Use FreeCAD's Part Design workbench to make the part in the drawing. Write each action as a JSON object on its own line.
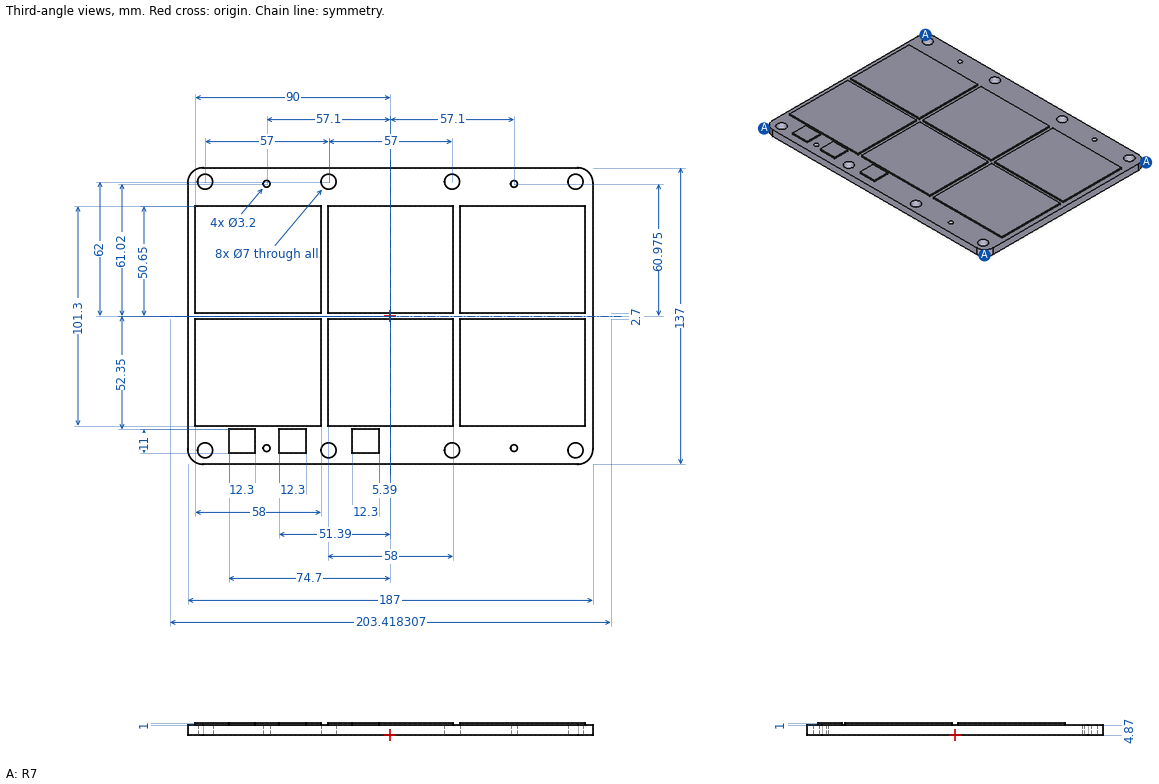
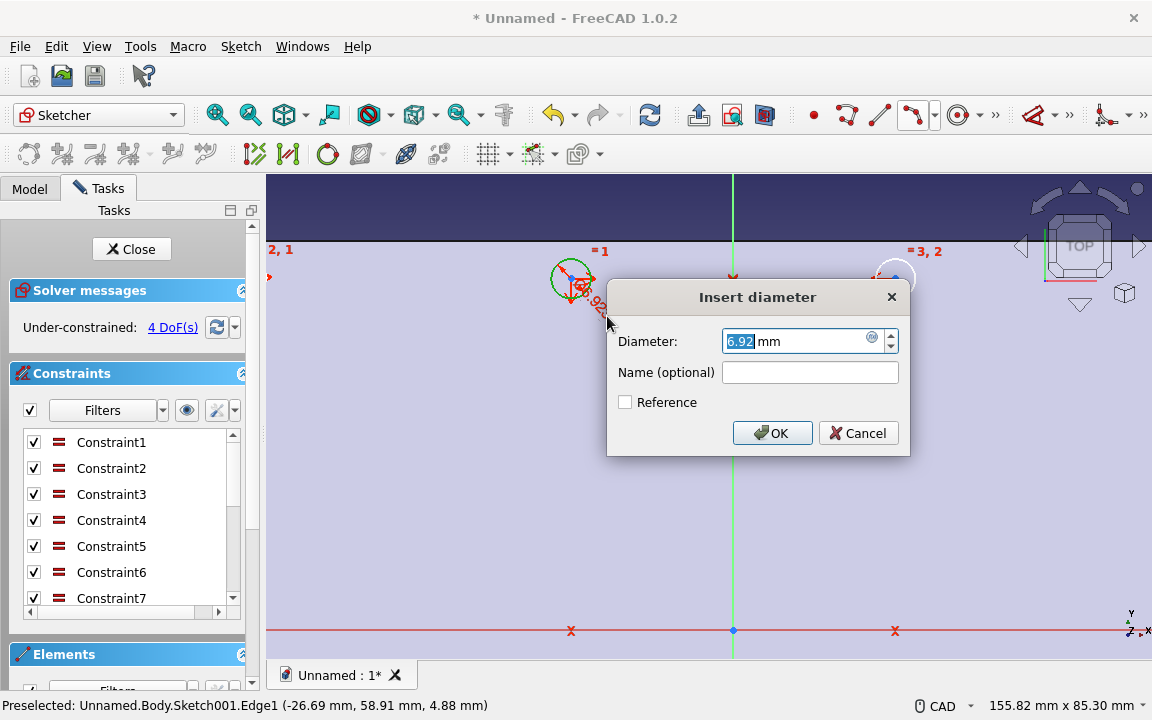
{"action": "type", "text": "7"}
{"action": "key", "text": "Return"}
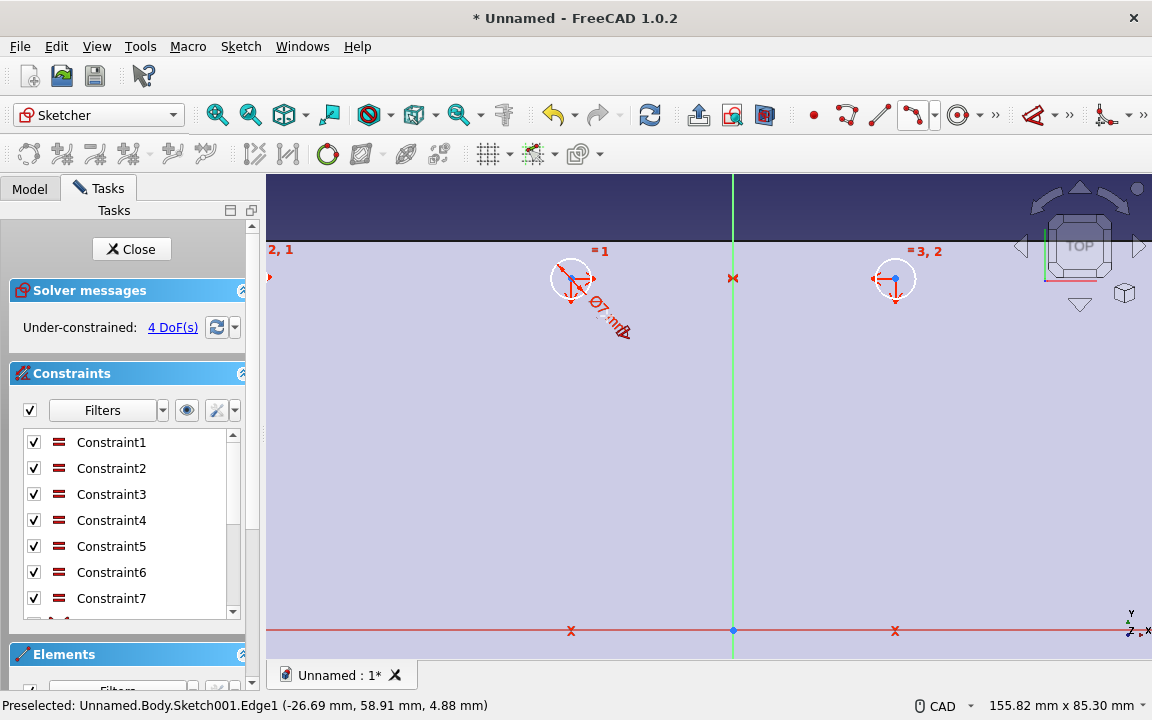
{"action": "left_click", "coordinate": [571, 279]}
{"action": "left_click", "coordinate": [537, 455]}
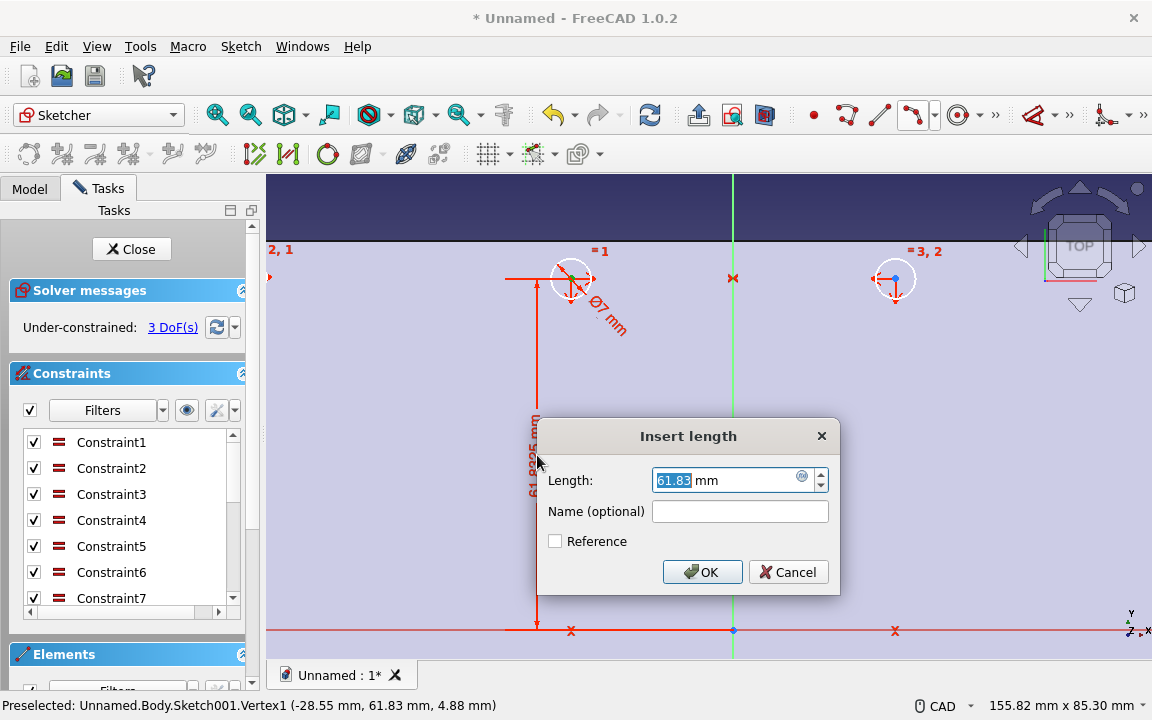
{"action": "type", "text": "62"}
{"action": "key", "text": "Return"}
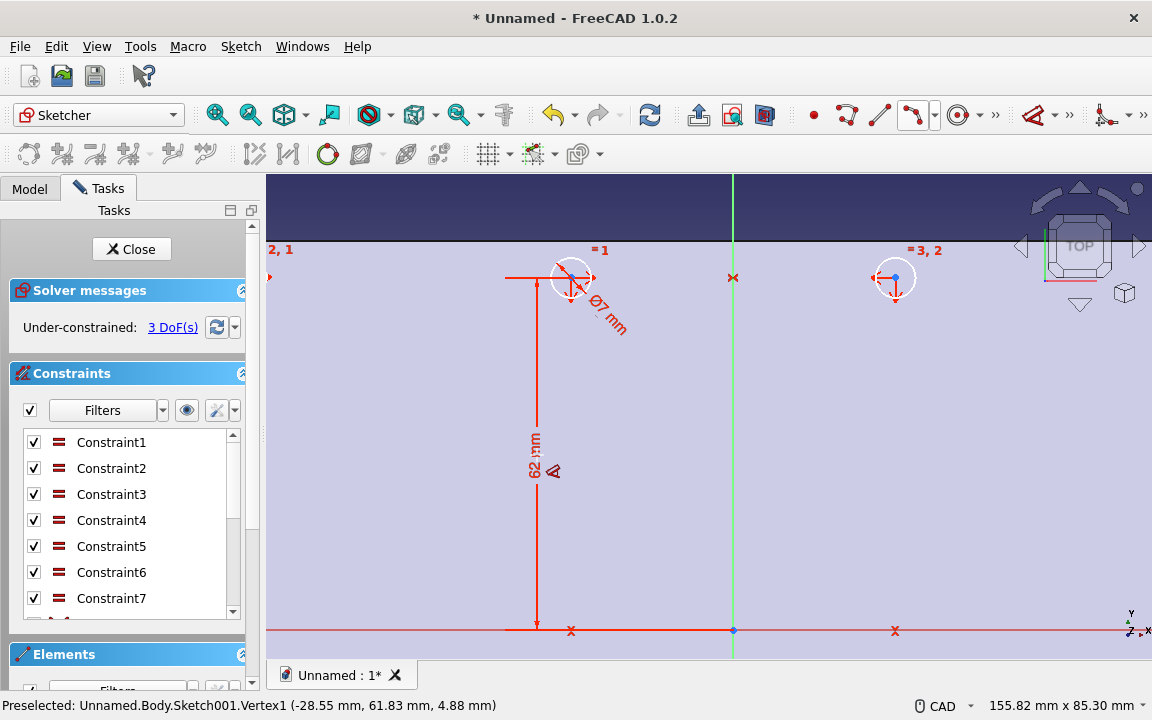
{"action": "scroll", "coordinate": [586, 292], "scroll_direction": "down", "scroll_amount": 5}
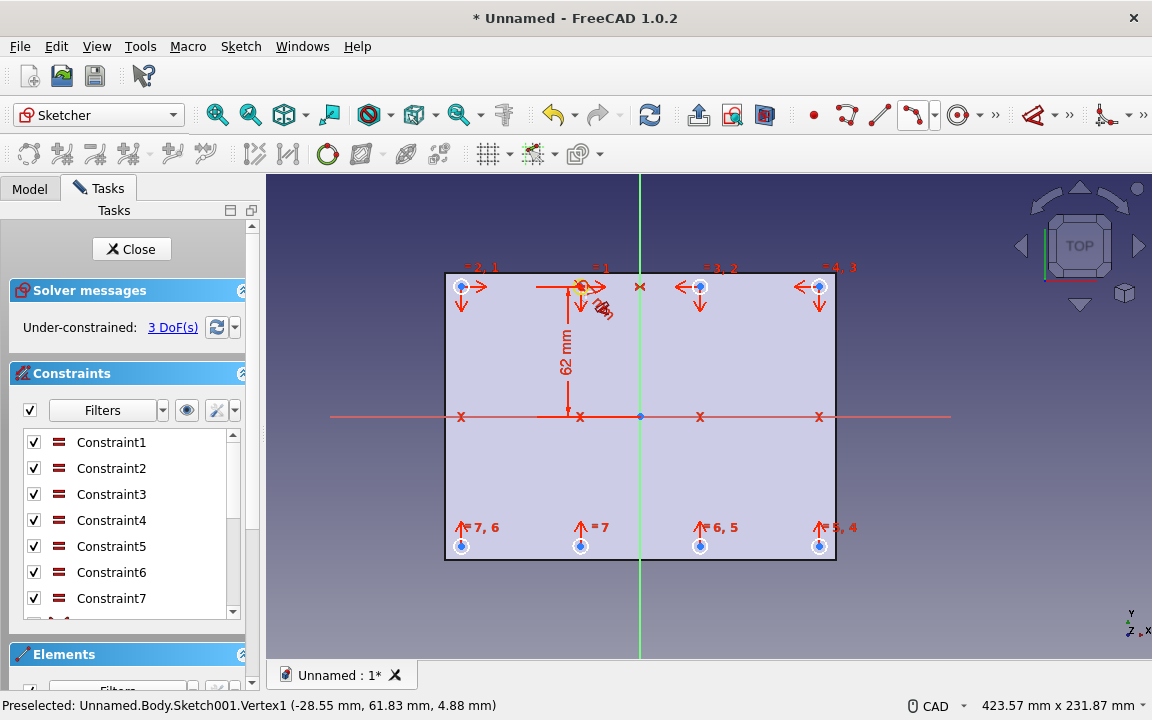
{"action": "left_click", "coordinate": [461, 287]}
{"action": "left_click", "coordinate": [427, 352]}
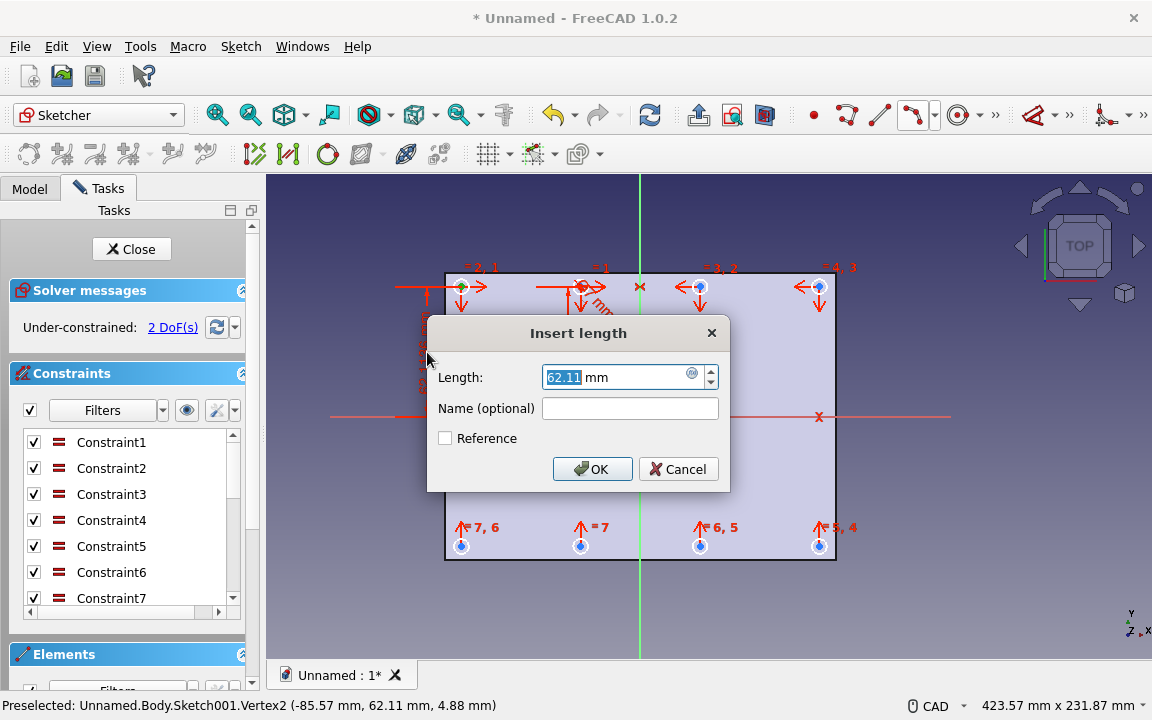
{"action": "type", "text": "62"}
{"action": "key", "text": "Return"}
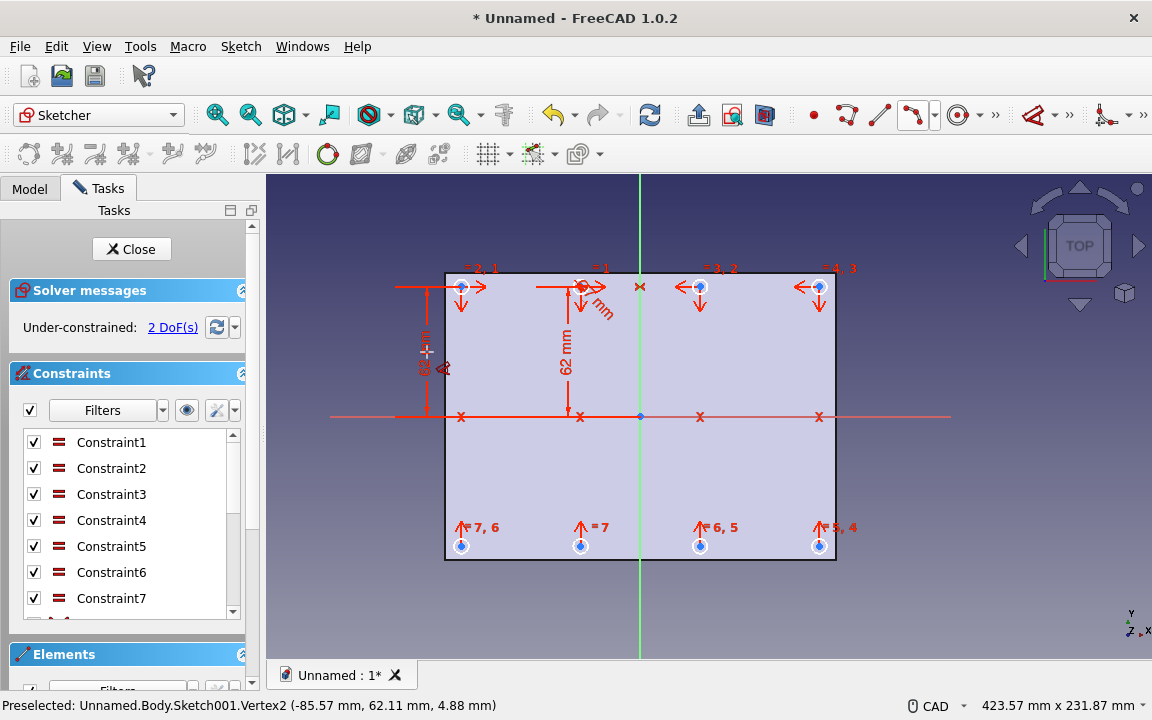
{"action": "left_click", "coordinate": [581, 287]}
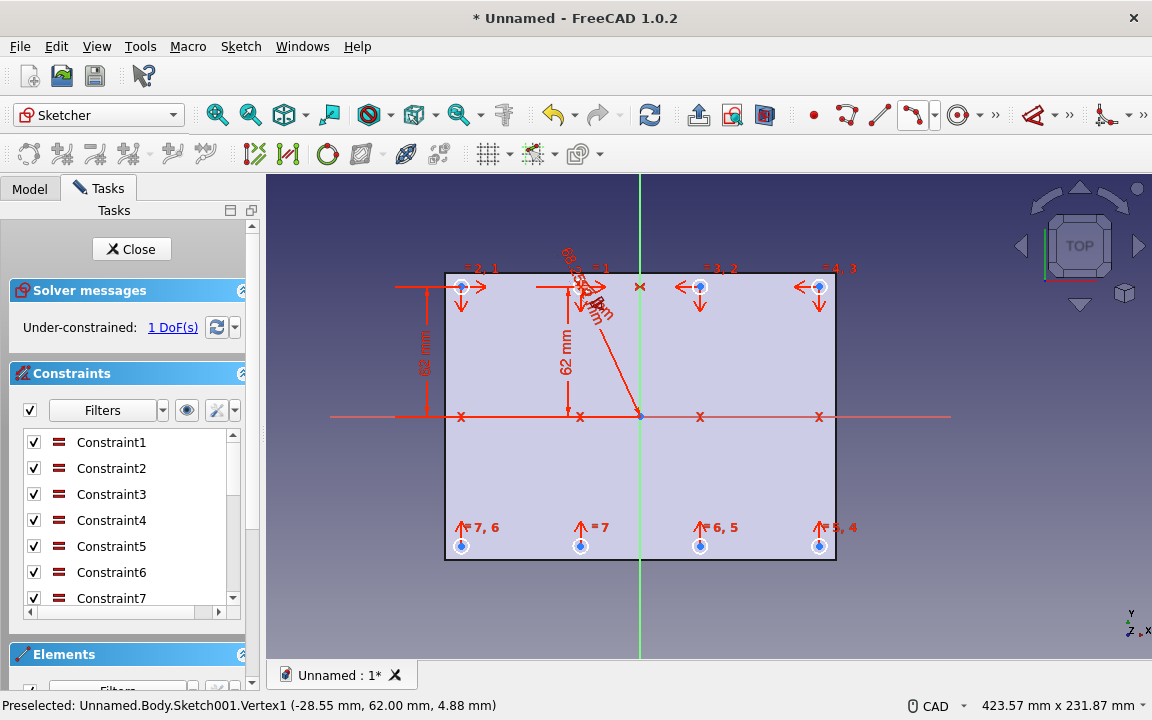
{"action": "left_click", "coordinate": [461, 287]}
{"action": "left_click", "coordinate": [521, 253]}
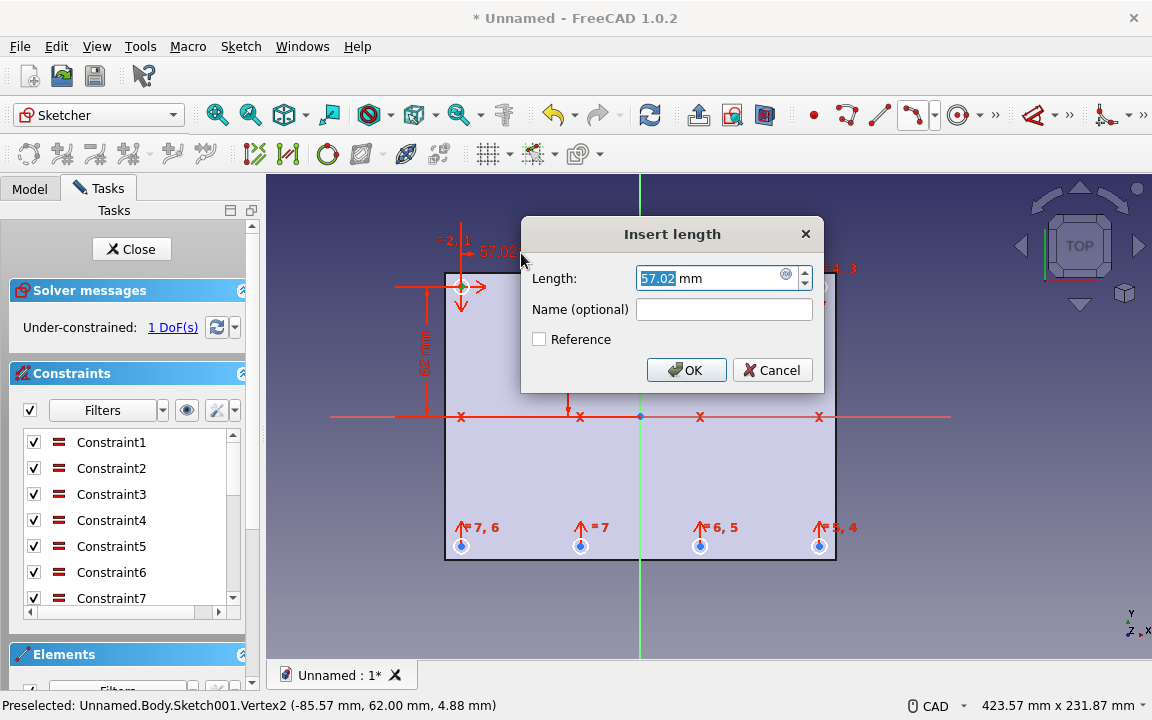
{"action": "type", "text": "57"}
{"action": "key", "text": "Return"}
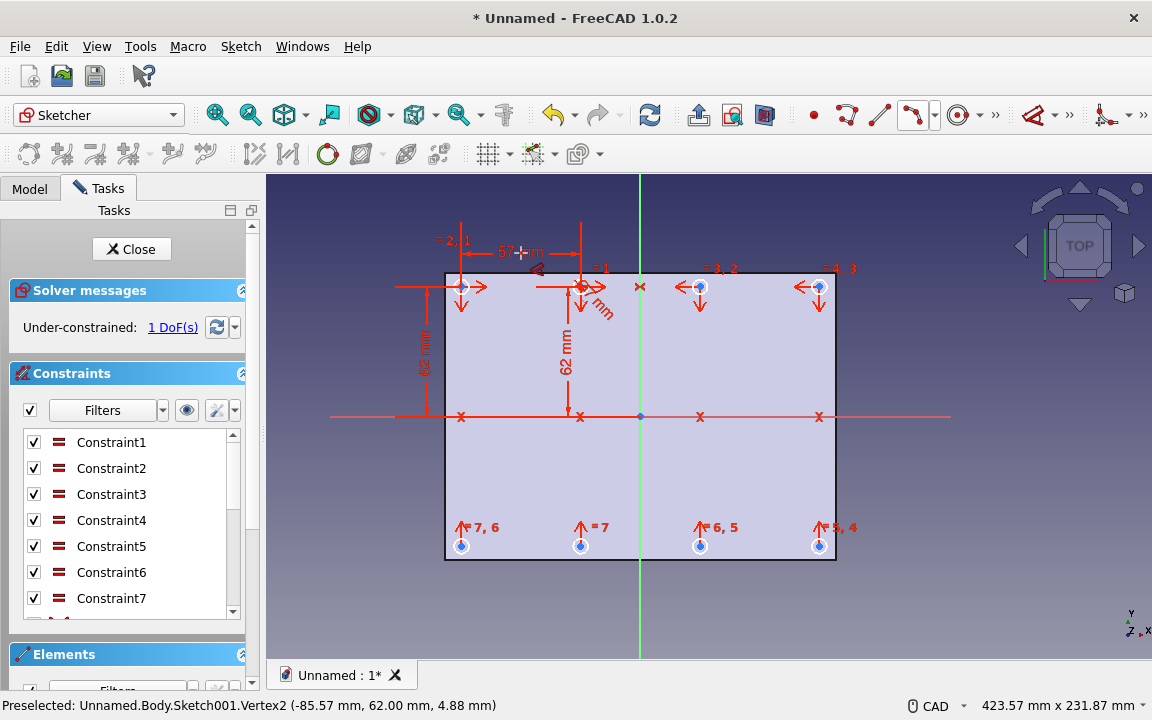
{"action": "left_click", "coordinate": [581, 287]}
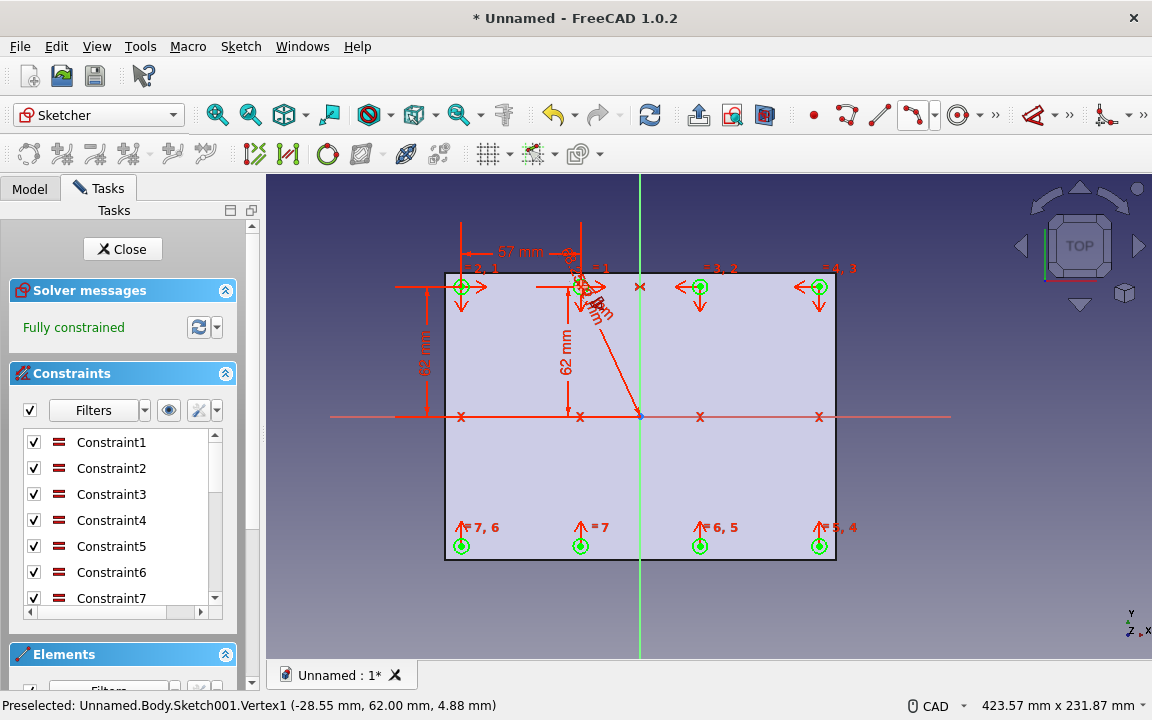
{"action": "left_click", "coordinate": [700, 287]}
{"action": "left_click", "coordinate": [613, 253]}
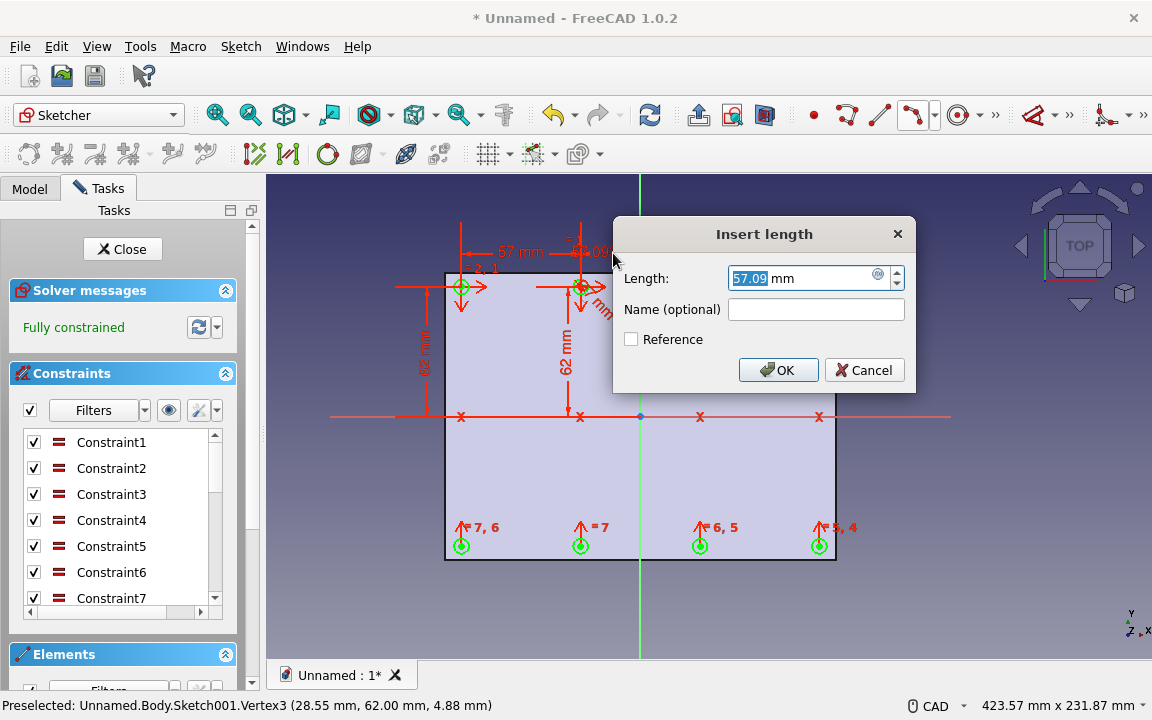
{"action": "type", "text": "57"}
{"action": "key", "text": "Return"}
{"action": "key", "text": "Escape"}